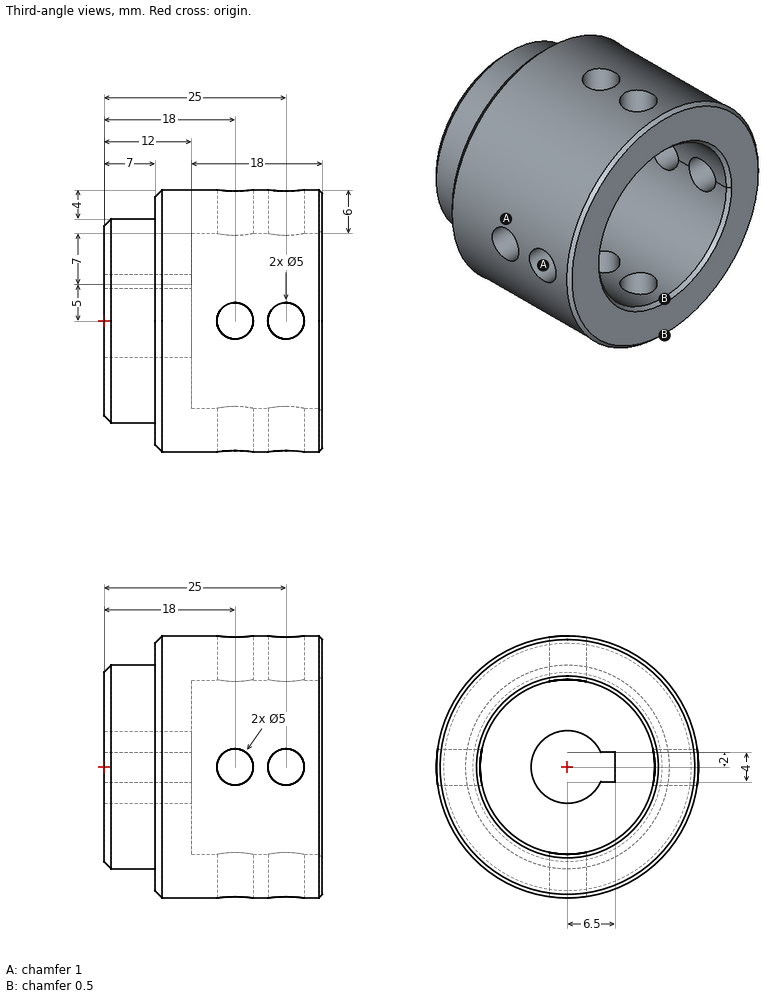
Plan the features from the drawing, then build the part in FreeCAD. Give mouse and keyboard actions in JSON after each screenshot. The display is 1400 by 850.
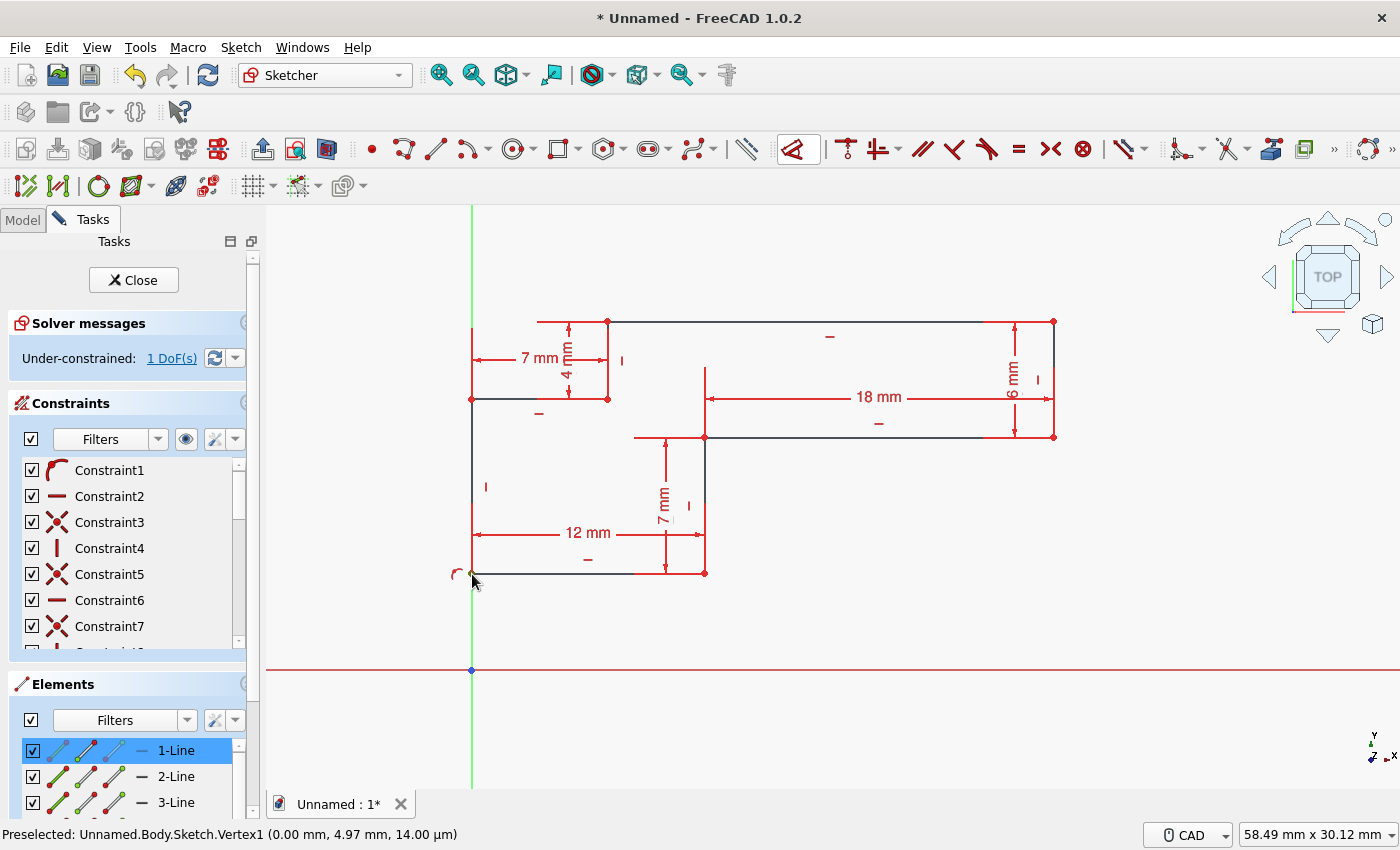
{"action": "key", "text": "i"}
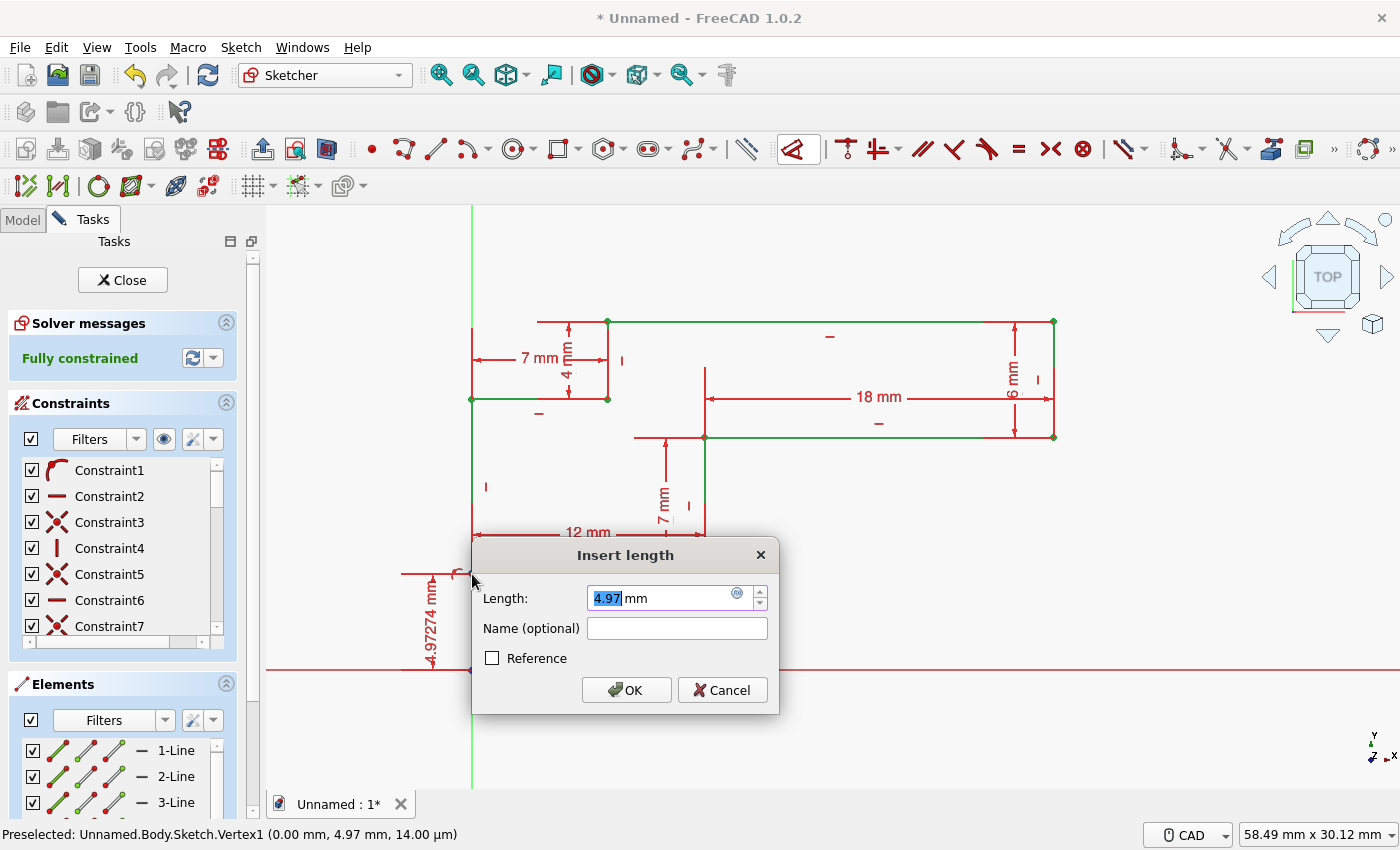
{"action": "type", "text": "5"}
{"action": "key", "text": "Return"}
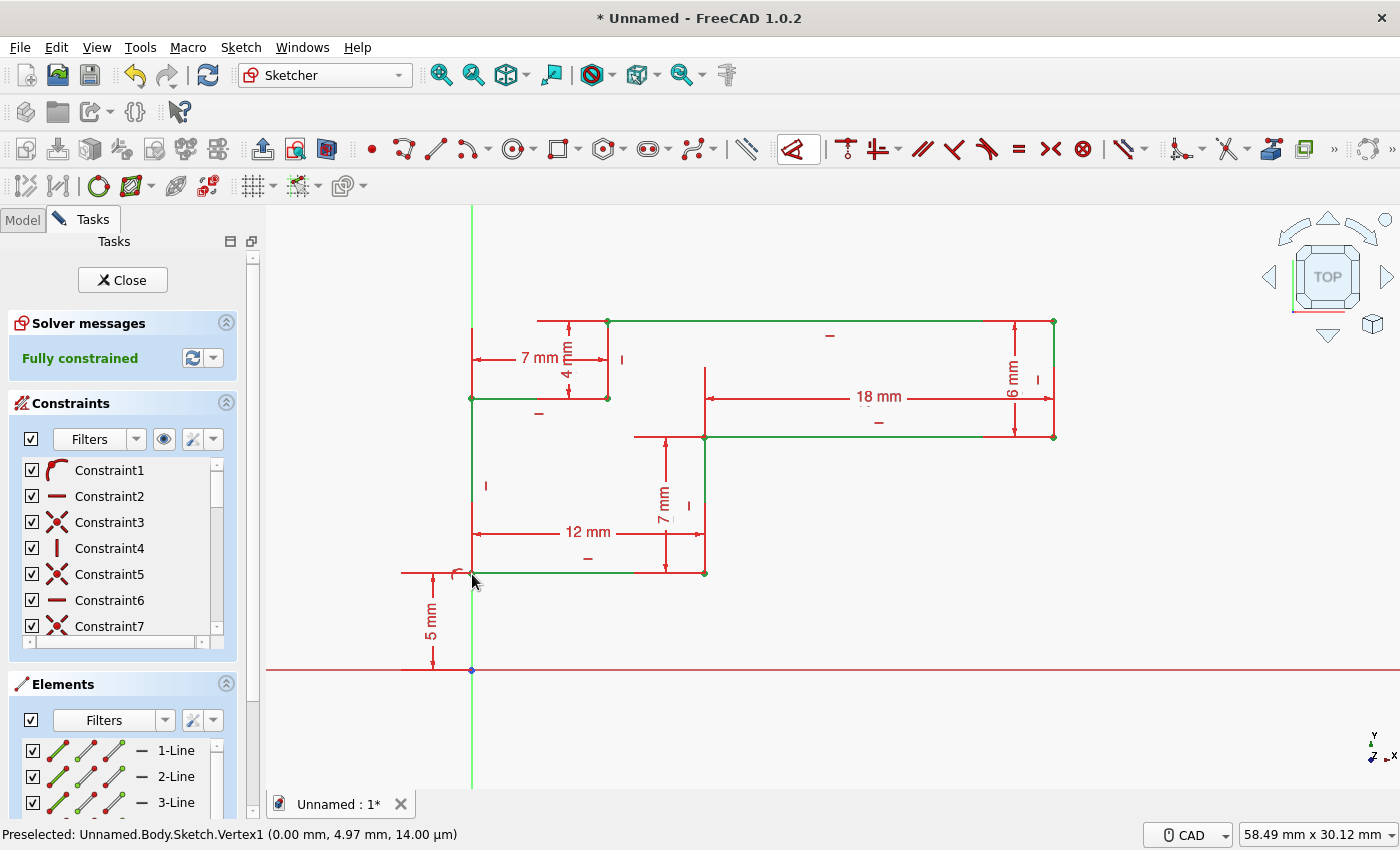
{"action": "left_click", "coordinate": [123, 280]}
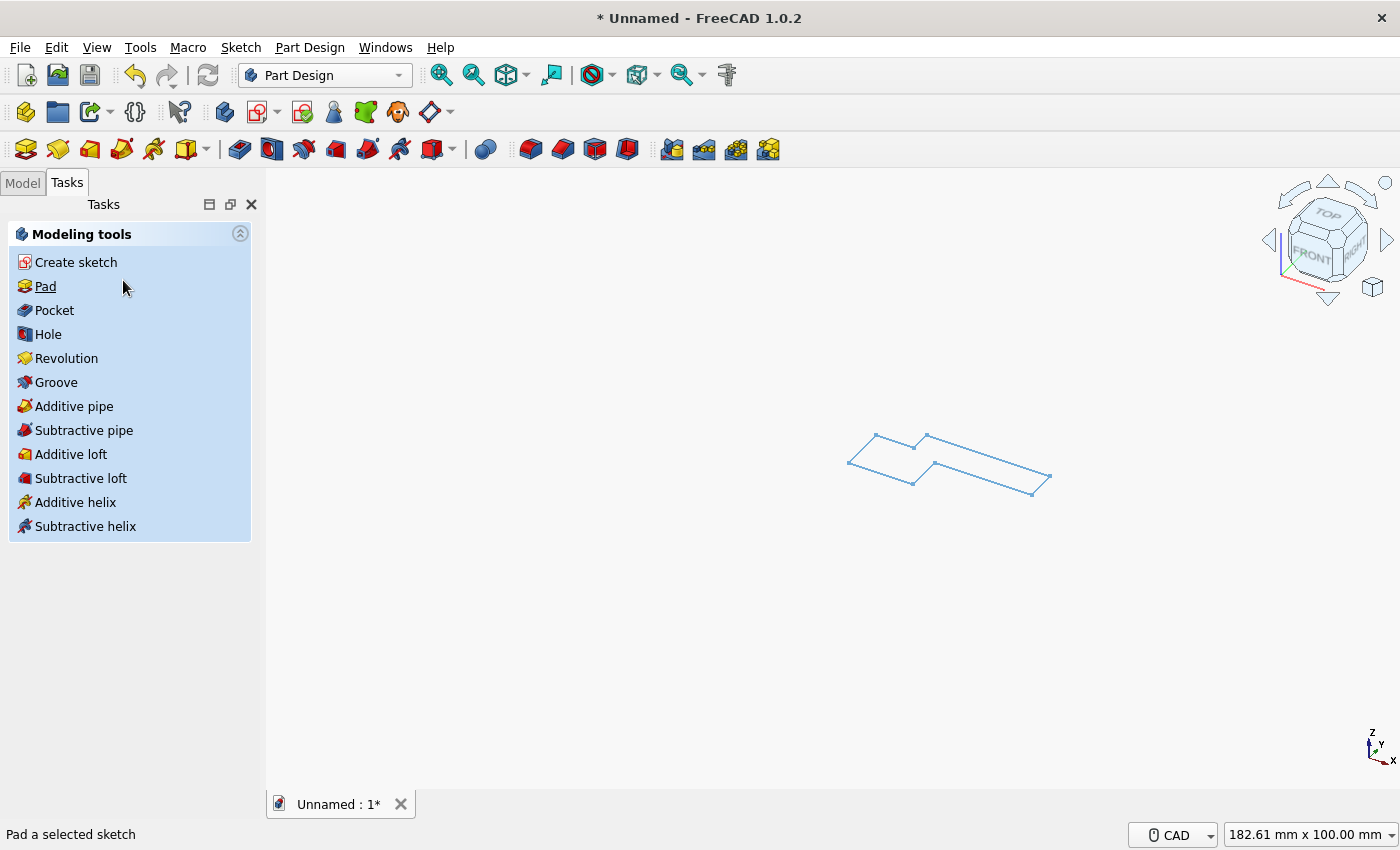
{"action": "left_click", "coordinate": [58, 150]}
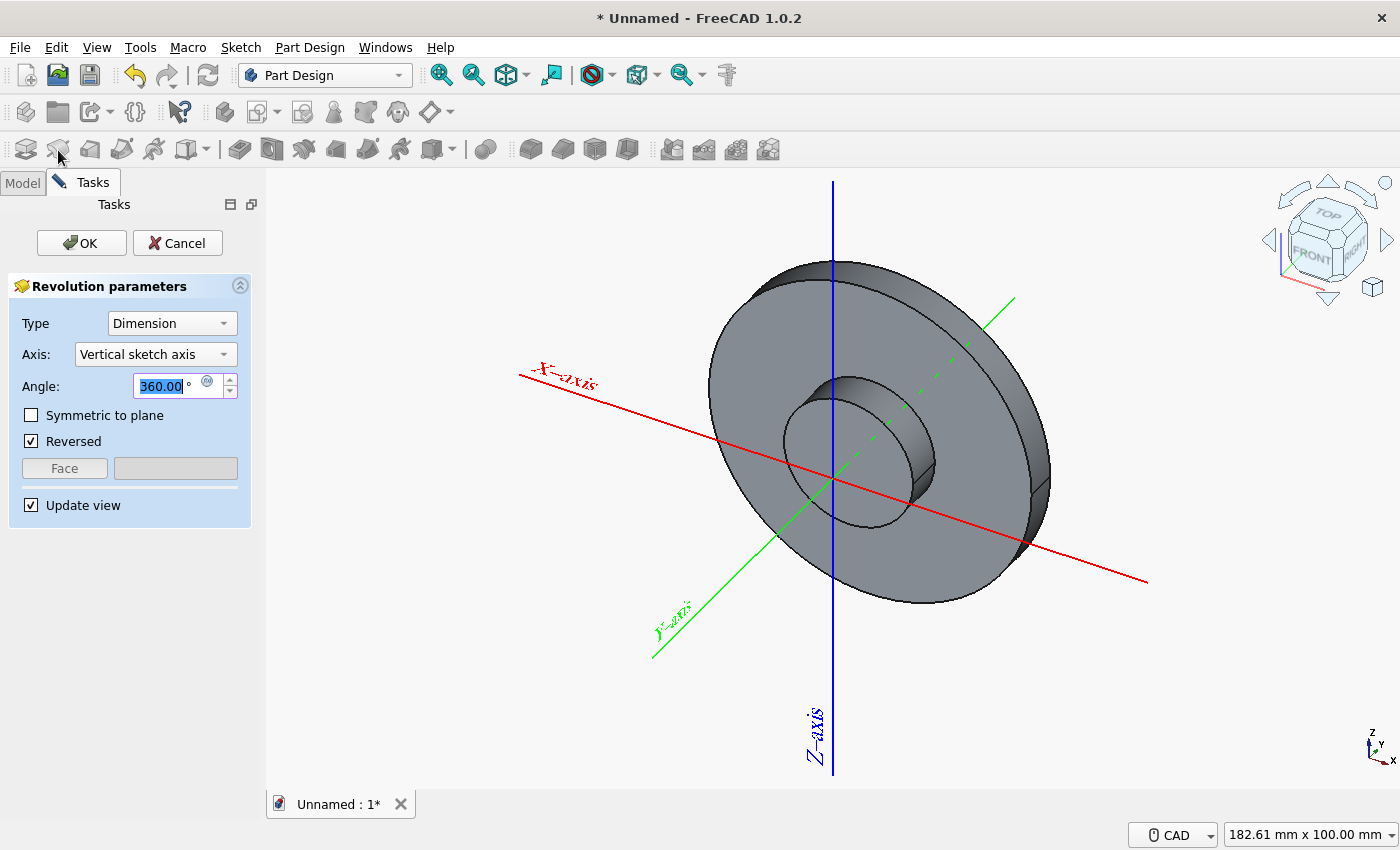
{"action": "left_click", "coordinate": [156, 354]}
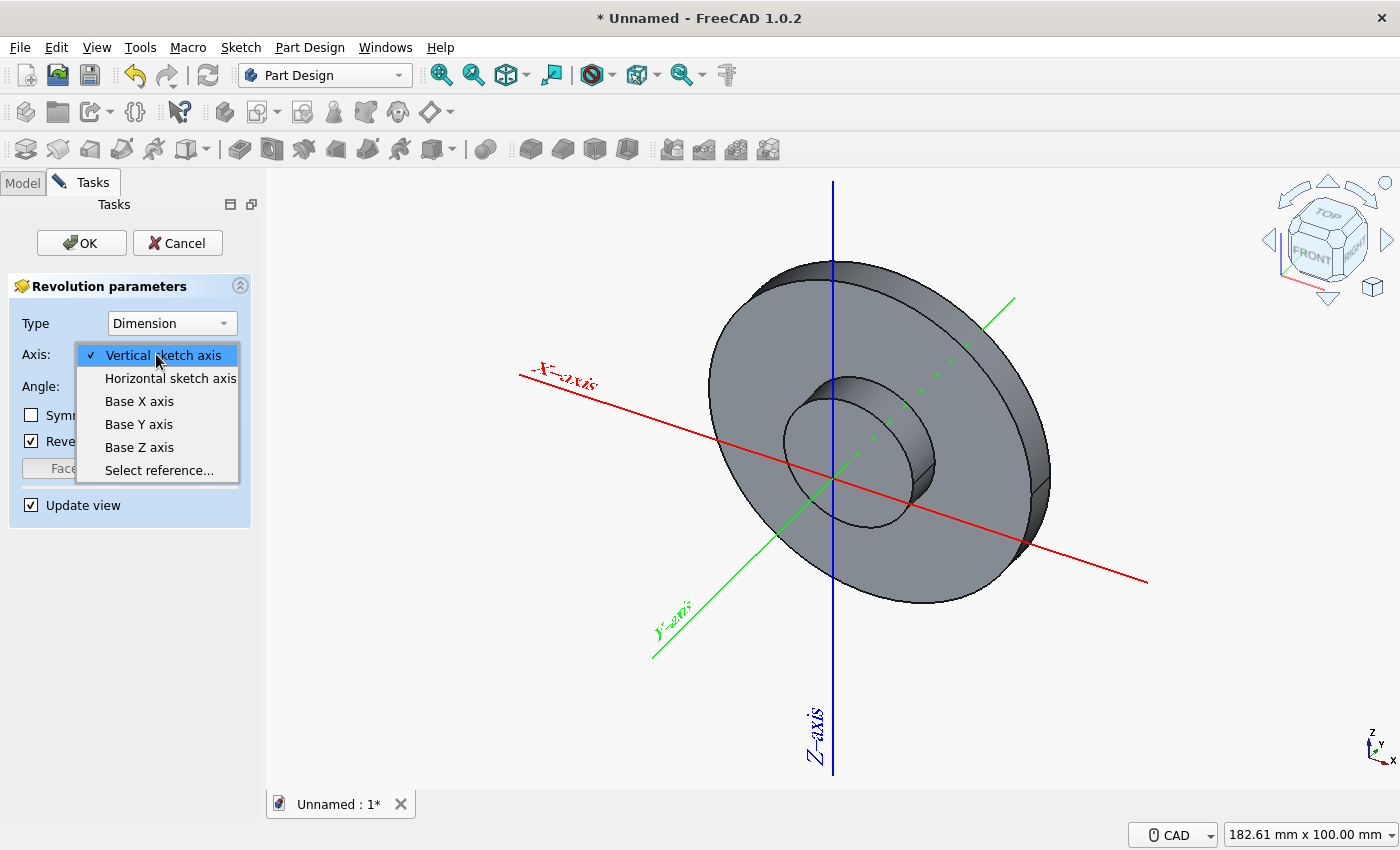
{"action": "left_click", "coordinate": [156, 378]}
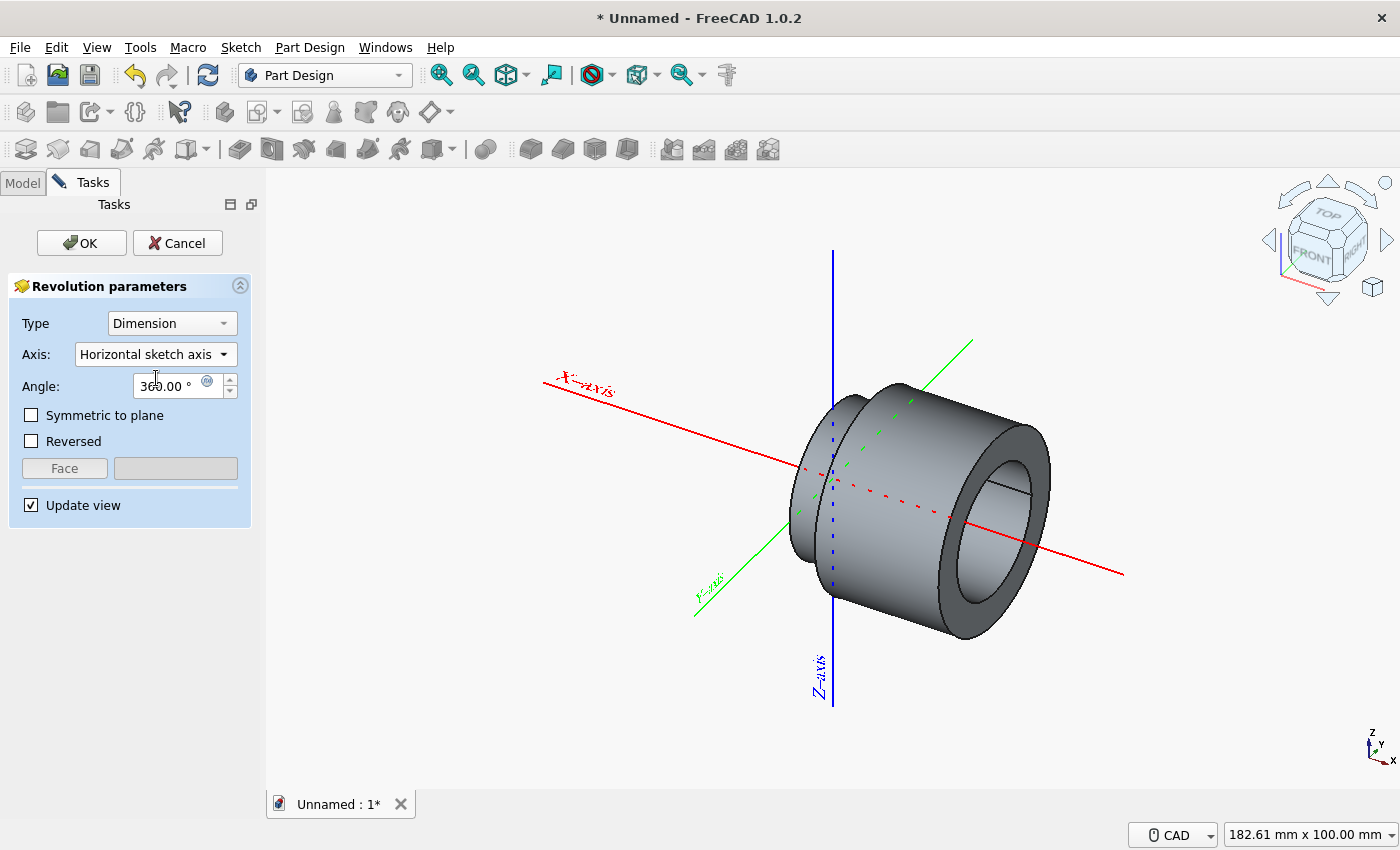
{"action": "left_click", "coordinate": [82, 243]}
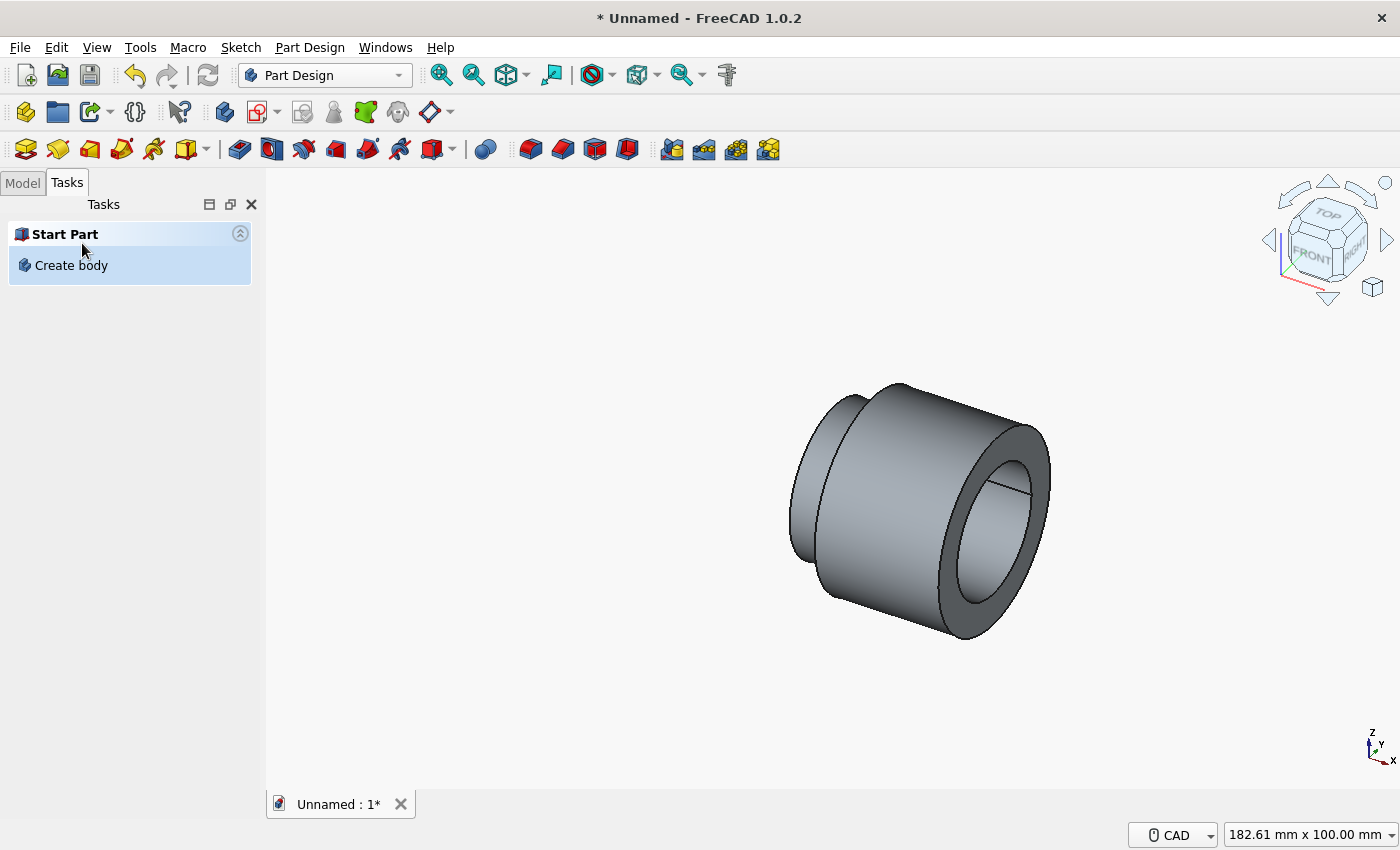
{"action": "left_click", "coordinate": [258, 112]}